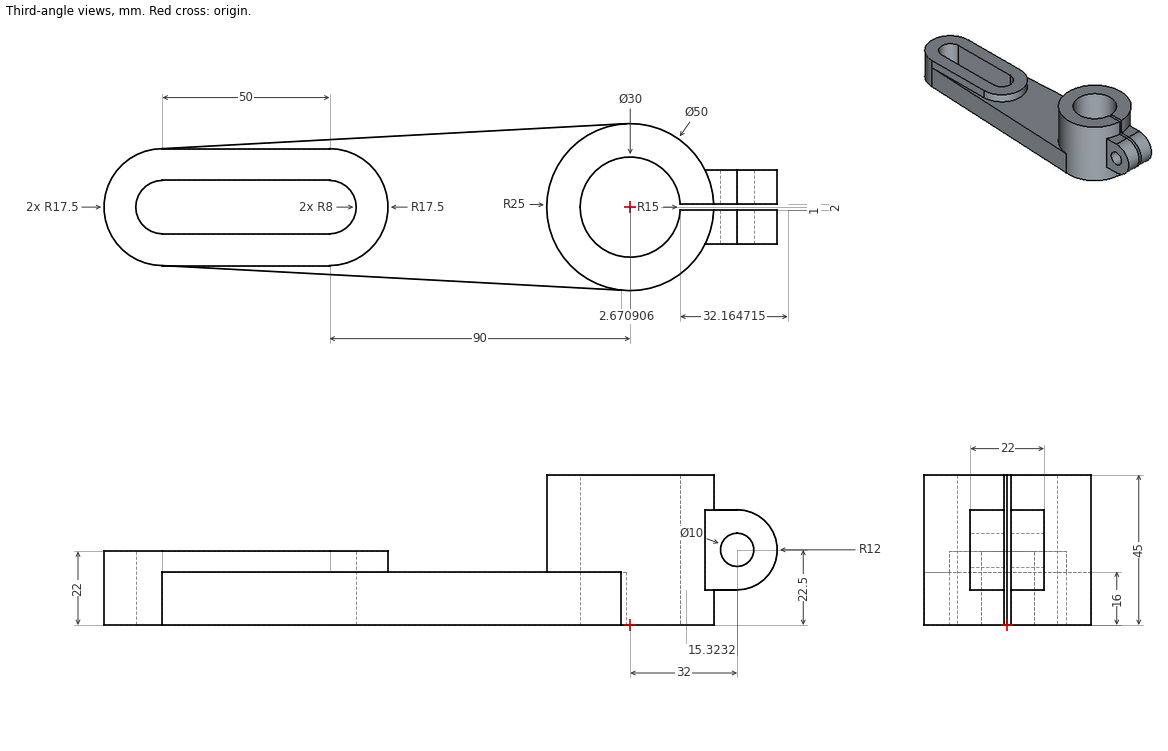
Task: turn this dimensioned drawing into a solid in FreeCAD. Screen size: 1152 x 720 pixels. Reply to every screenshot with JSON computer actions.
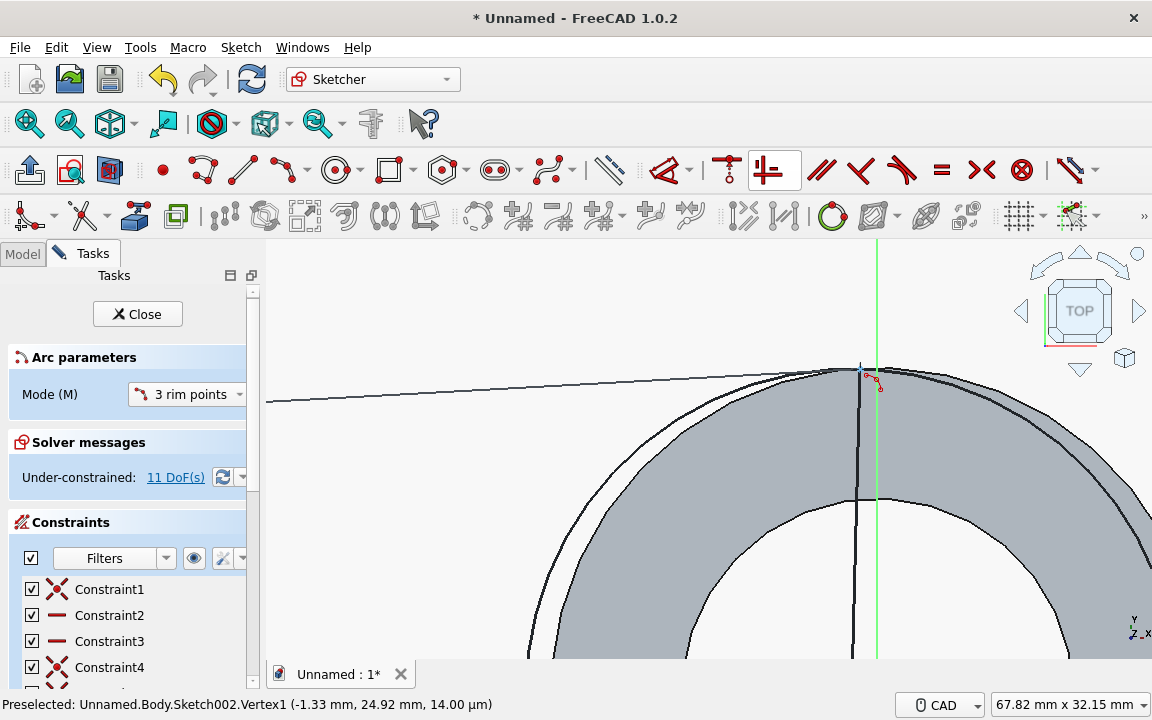
{"action": "scroll", "coordinate": [862, 369], "scroll_direction": "down", "scroll_amount": 7}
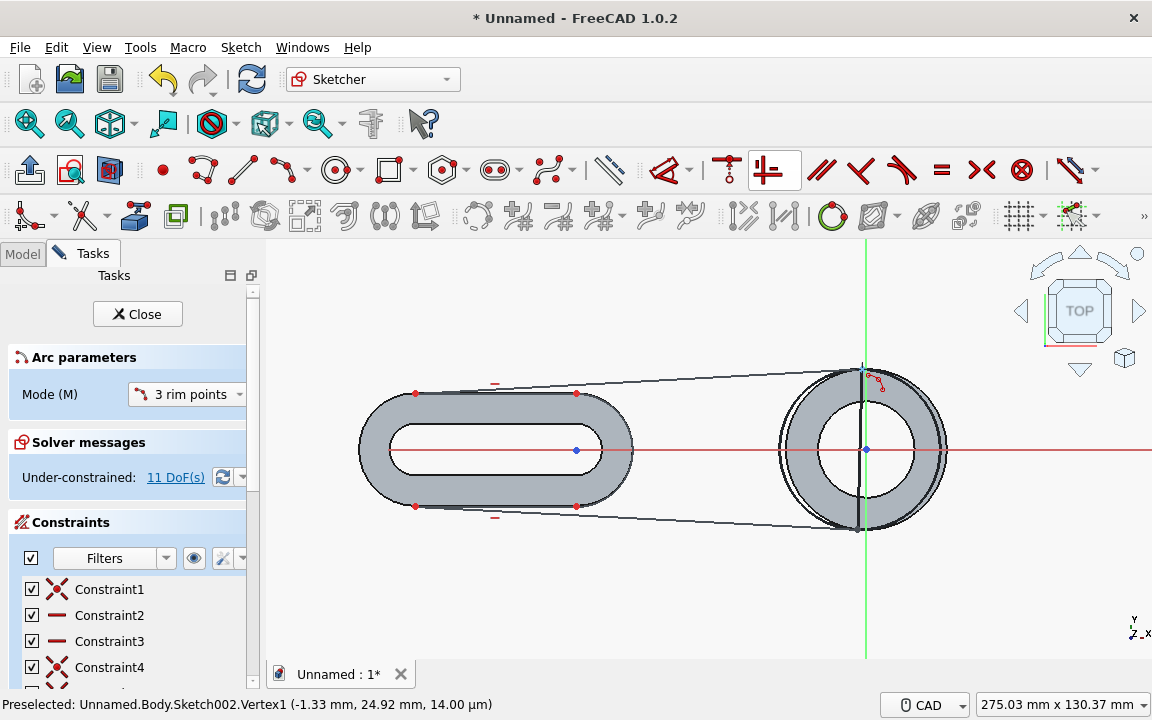
{"action": "left_click", "coordinate": [790, 424]}
{"action": "key", "text": "Escape"}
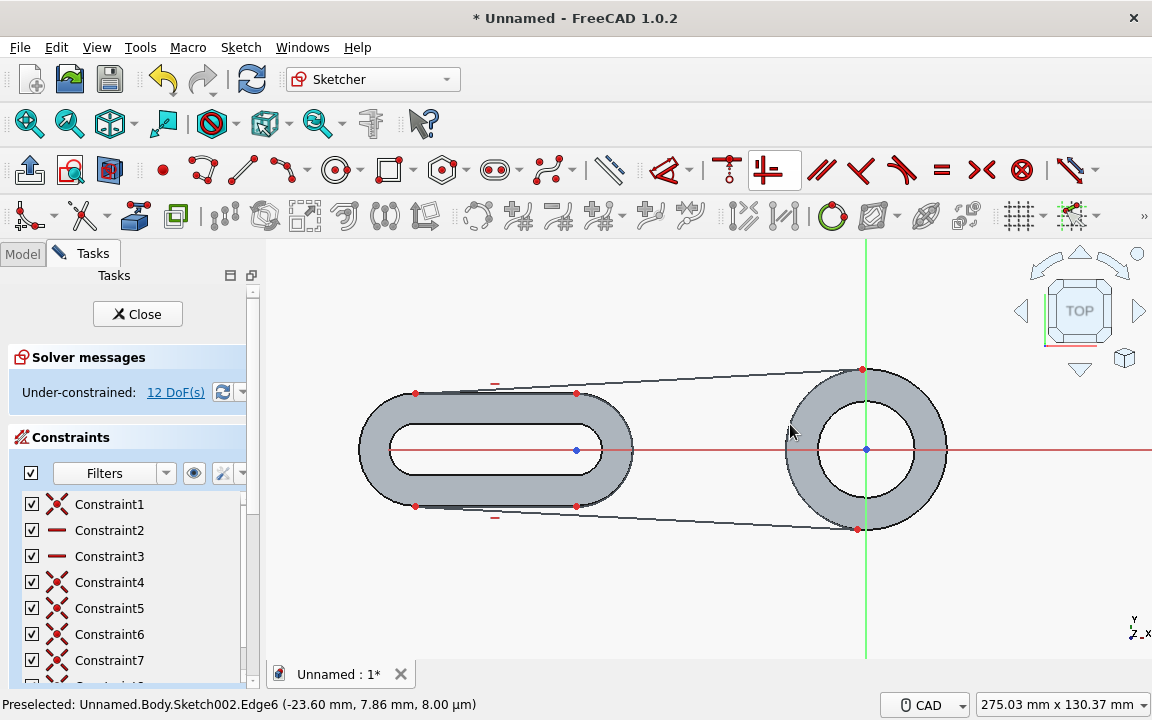
{"action": "left_click", "coordinate": [728, 377]}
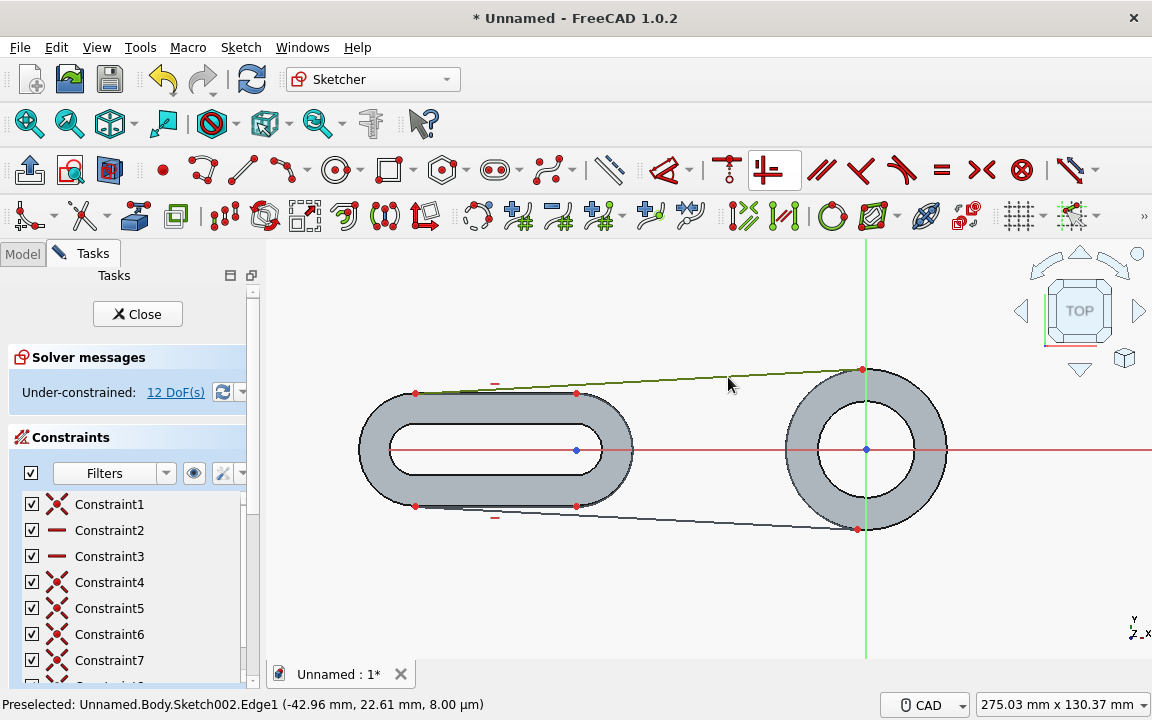
{"action": "left_click", "coordinate": [801, 403]}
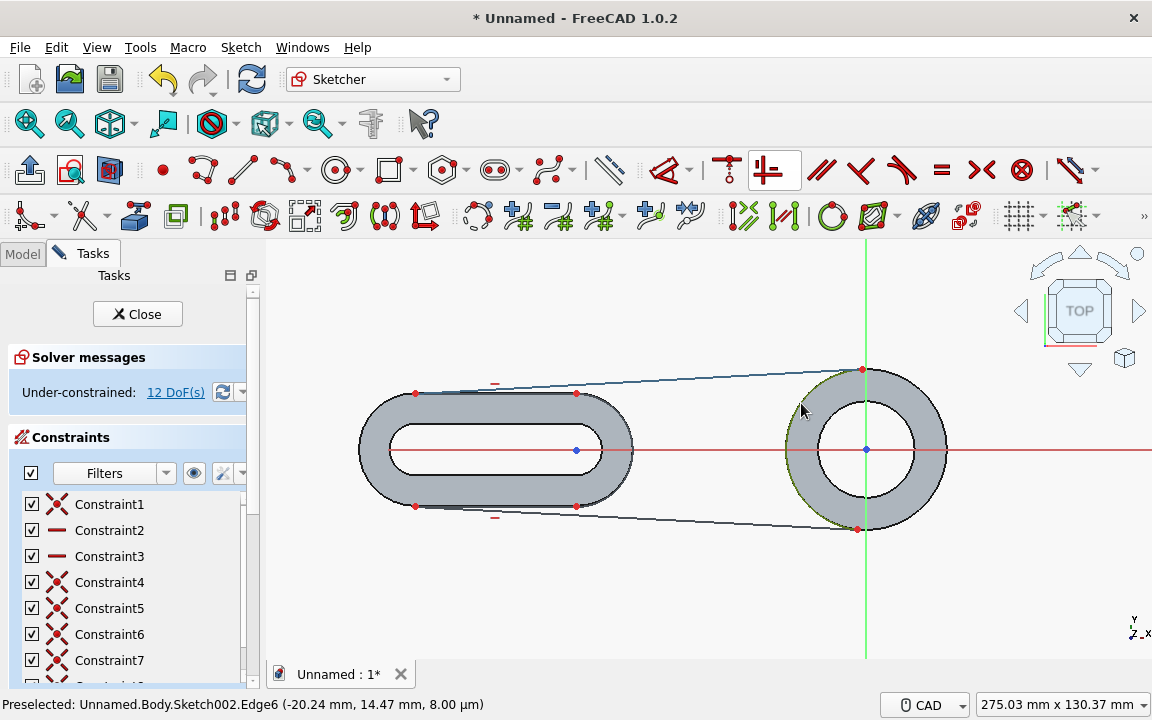
{"action": "key", "text": "t"}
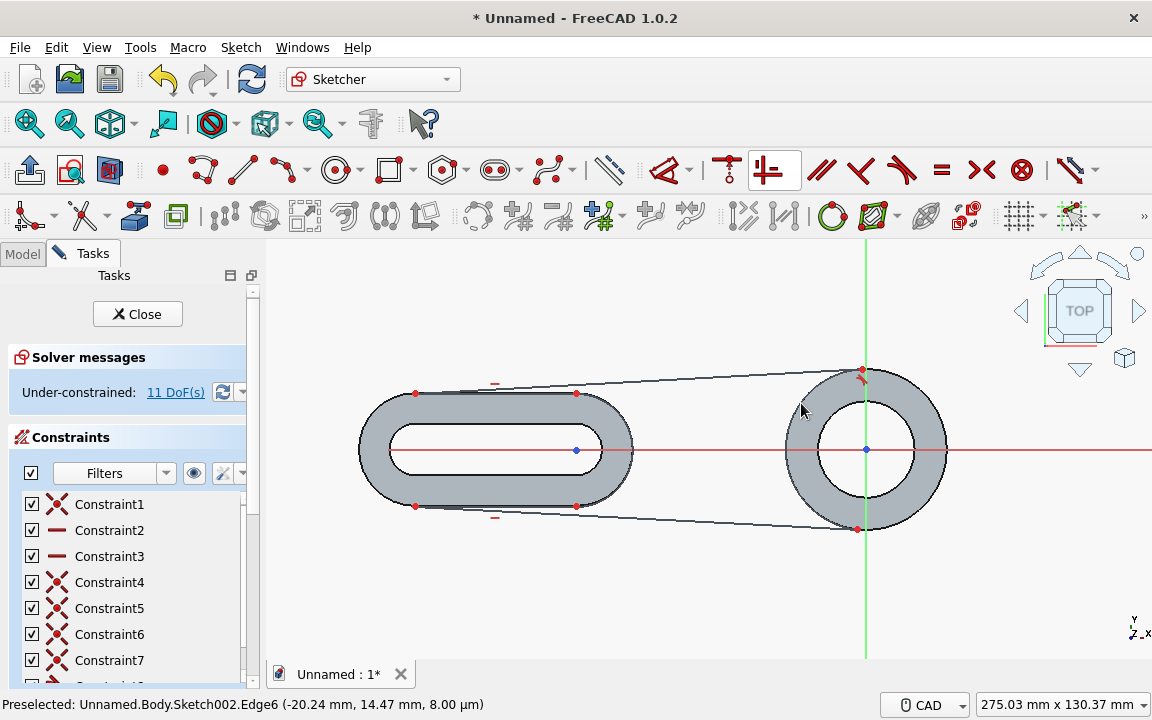
{"action": "scroll", "coordinate": [544, 394], "scroll_direction": "up", "scroll_amount": 4}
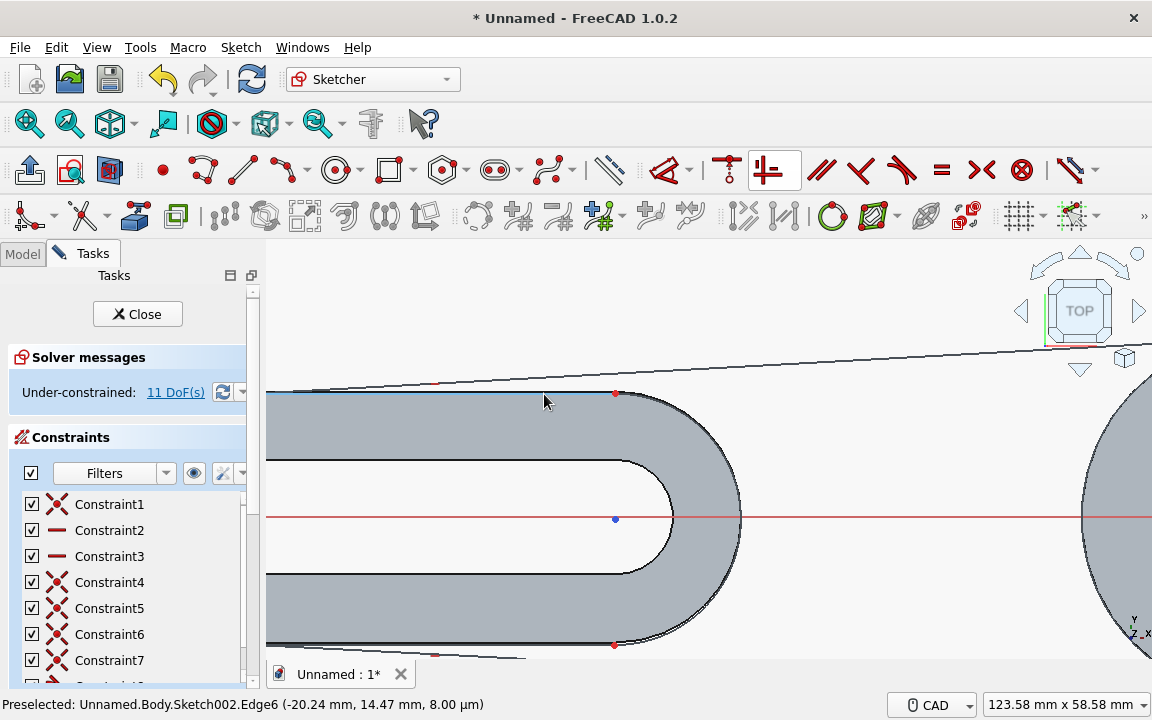
{"action": "left_click", "coordinate": [544, 394]}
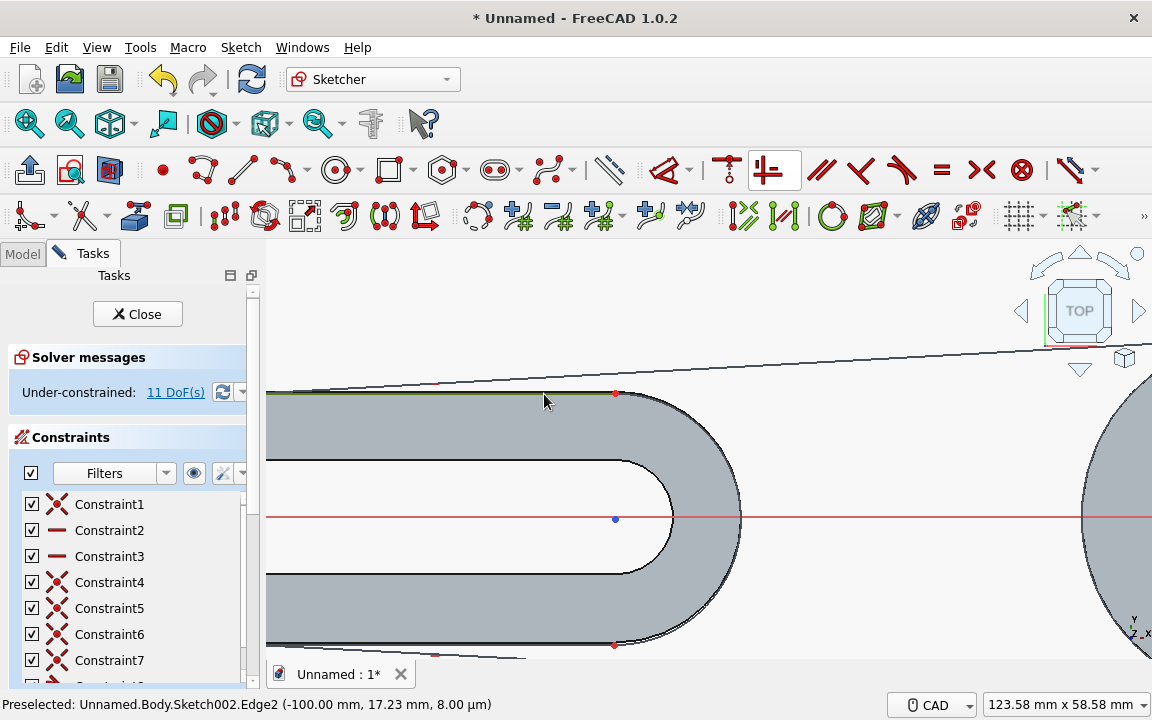
{"action": "left_click", "coordinate": [717, 593]}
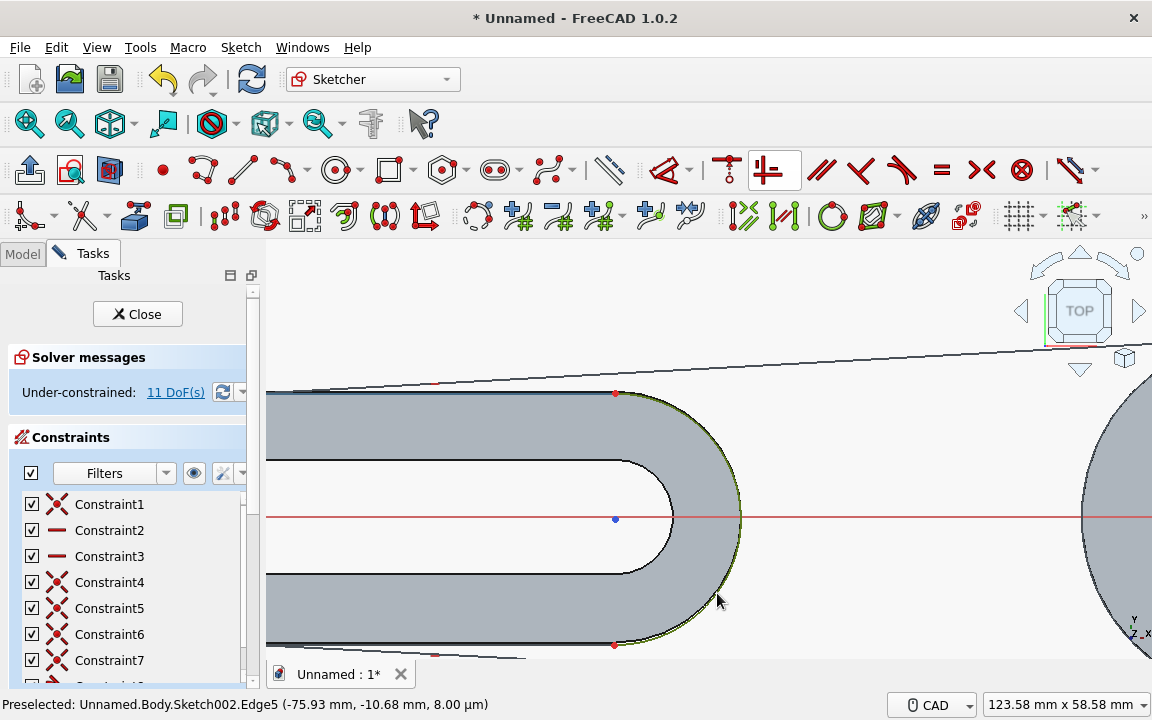
{"action": "left_click", "coordinate": [902, 170]}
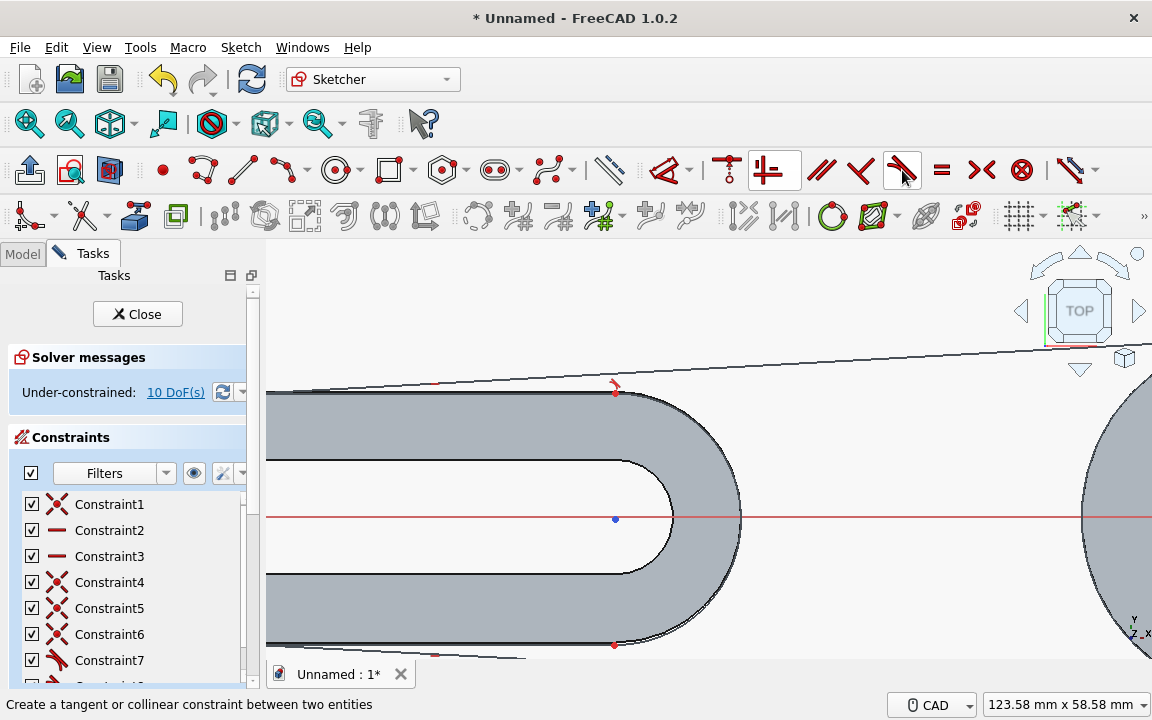
{"action": "scroll", "coordinate": [544, 394], "scroll_direction": "down", "scroll_amount": 4}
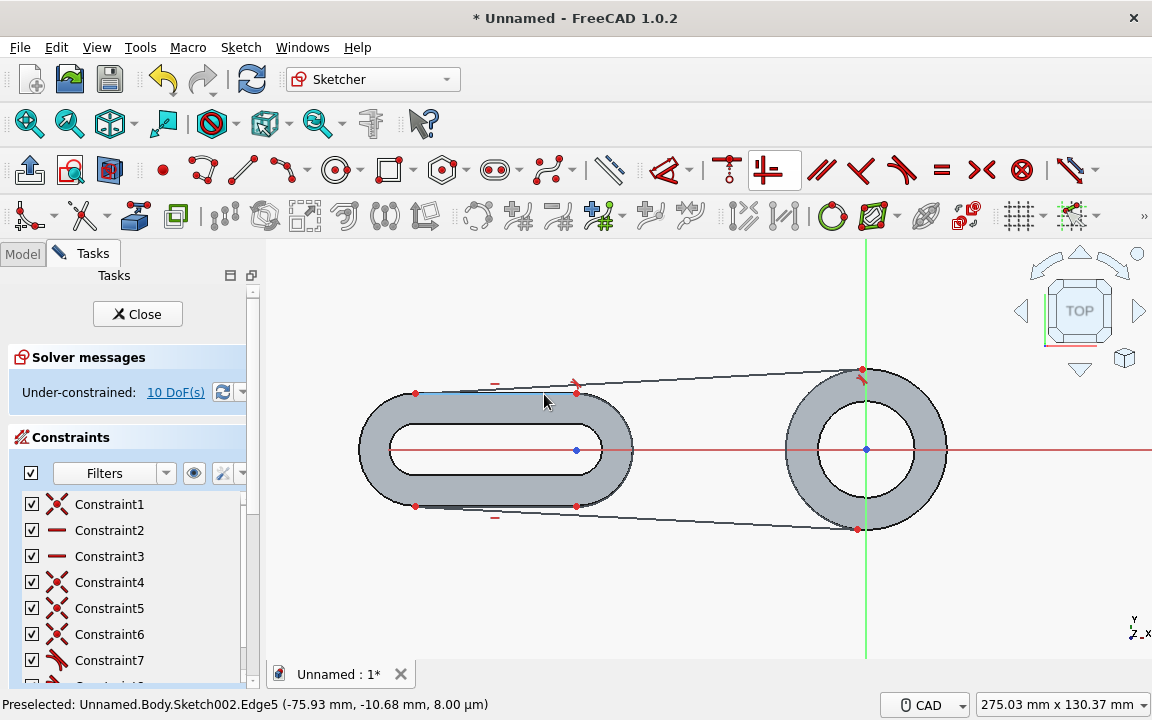
{"action": "scroll", "coordinate": [528, 507], "scroll_direction": "up", "scroll_amount": 5}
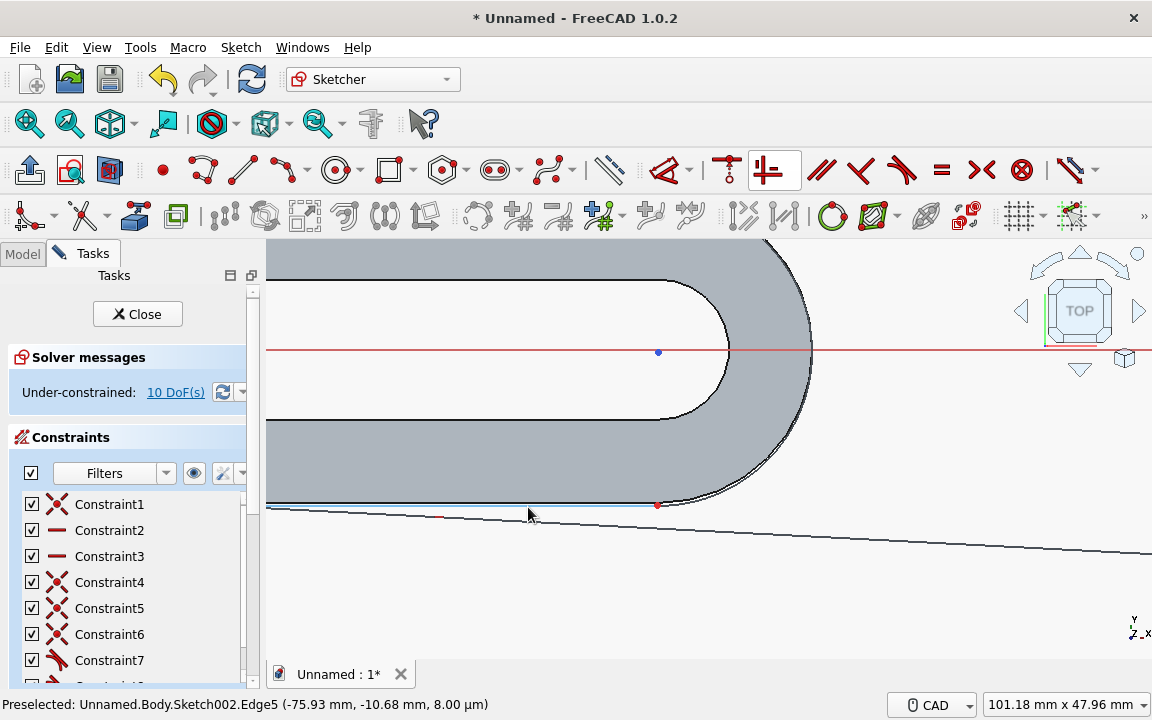
{"action": "left_click", "coordinate": [527, 506]}